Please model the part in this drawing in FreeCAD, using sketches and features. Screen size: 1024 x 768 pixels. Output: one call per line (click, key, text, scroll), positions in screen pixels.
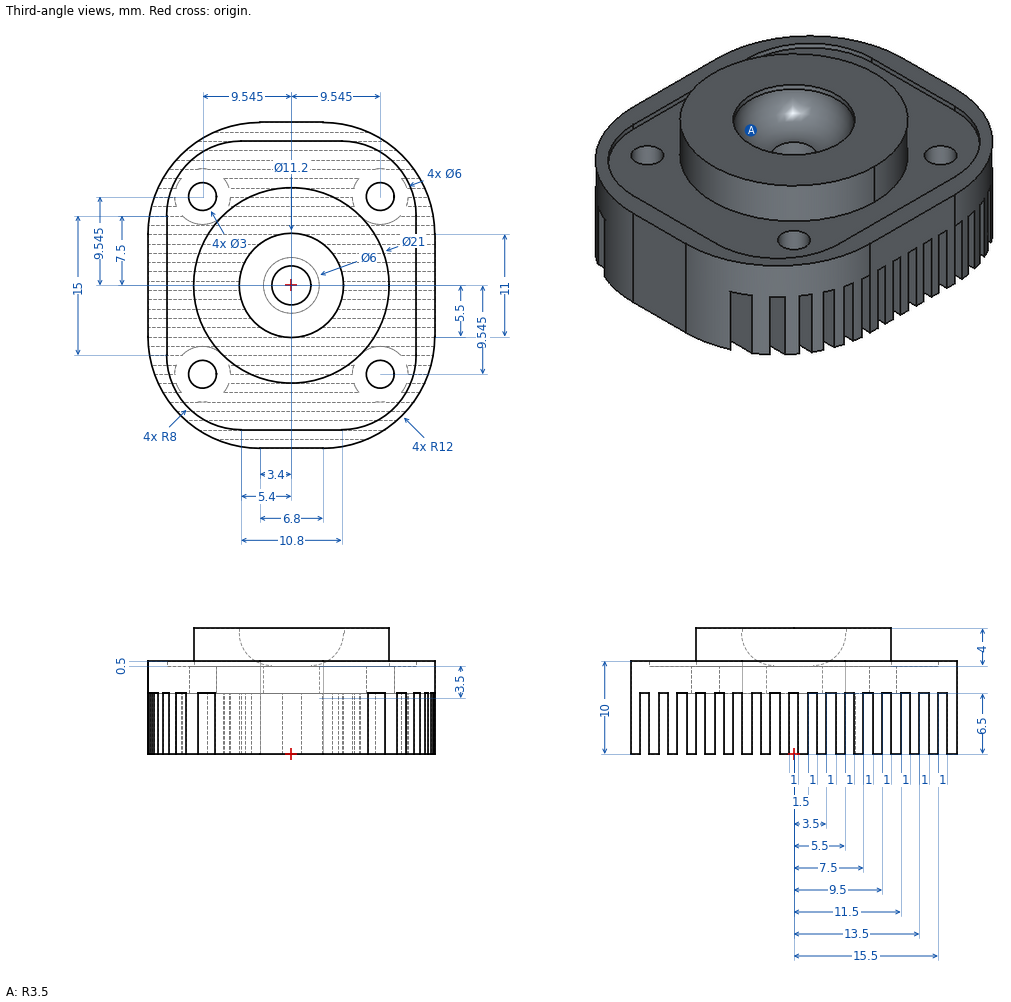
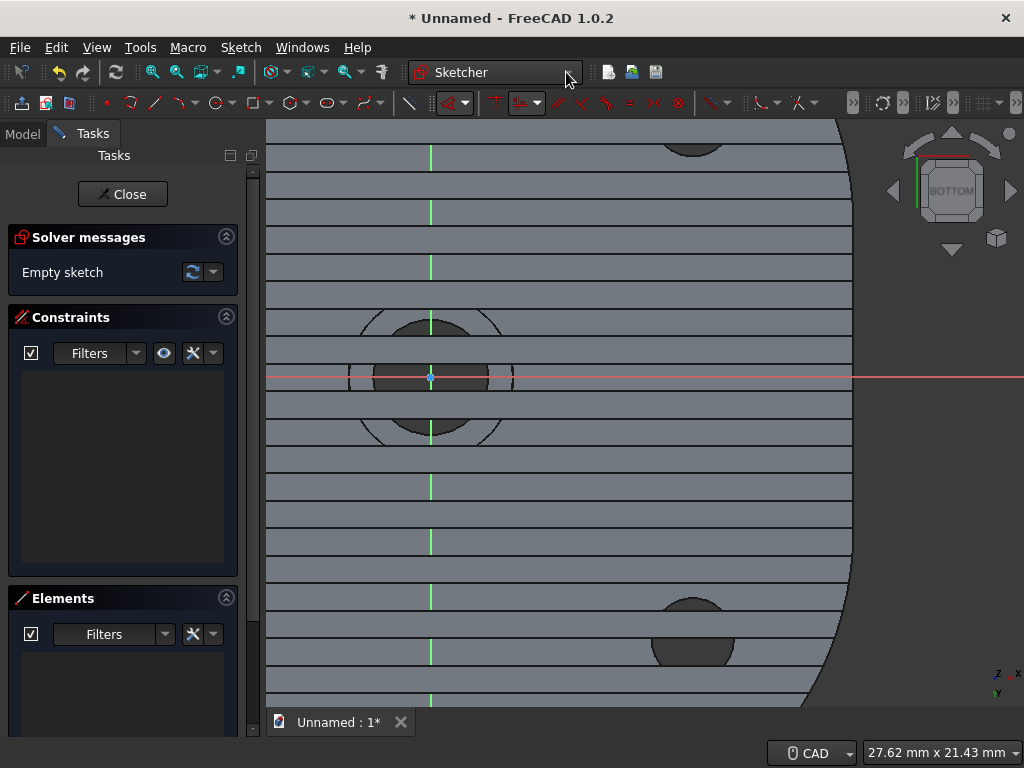
click(70, 104)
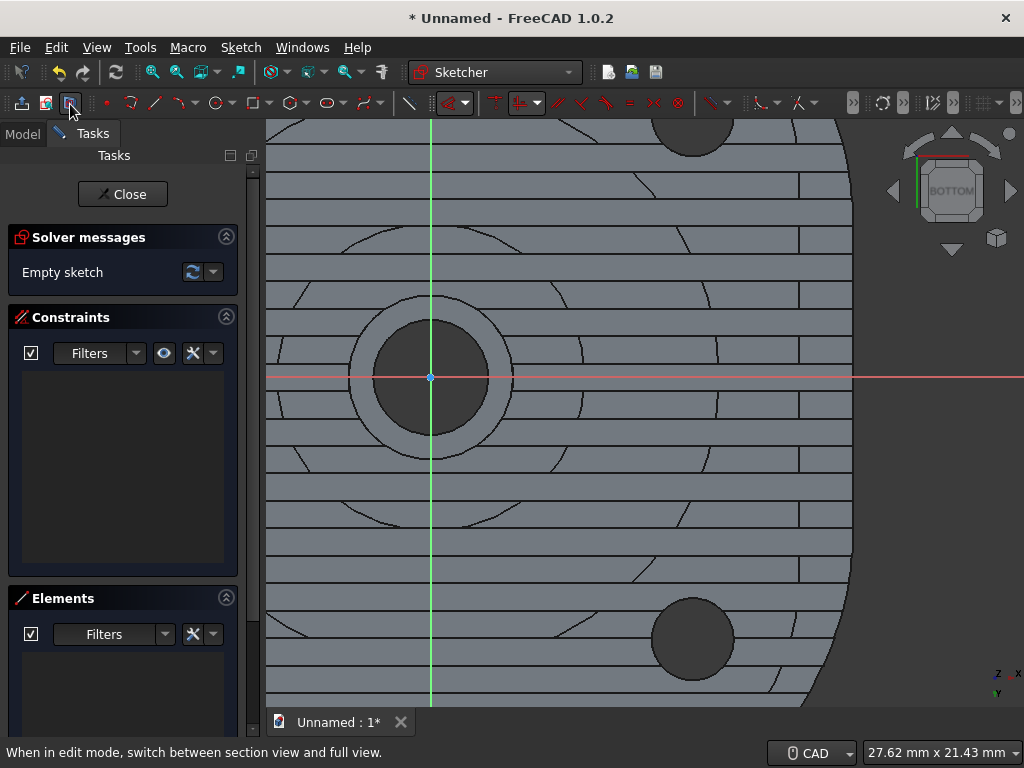
scroll(859, 574, down, 1)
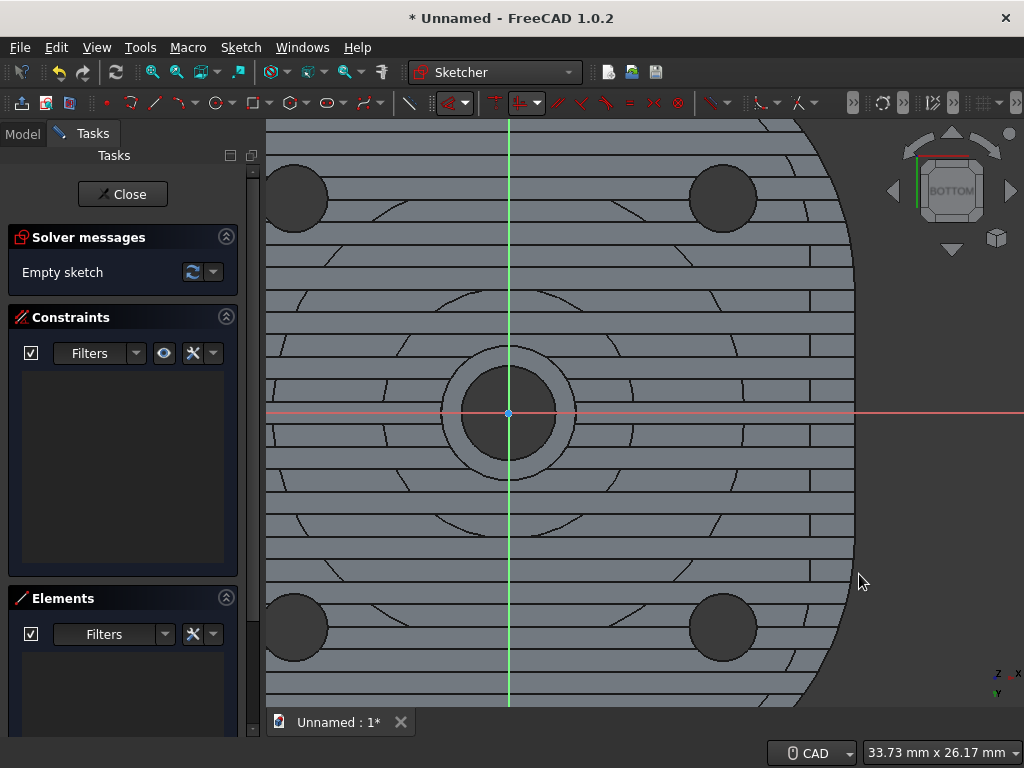
scroll(370, 413, up, 2)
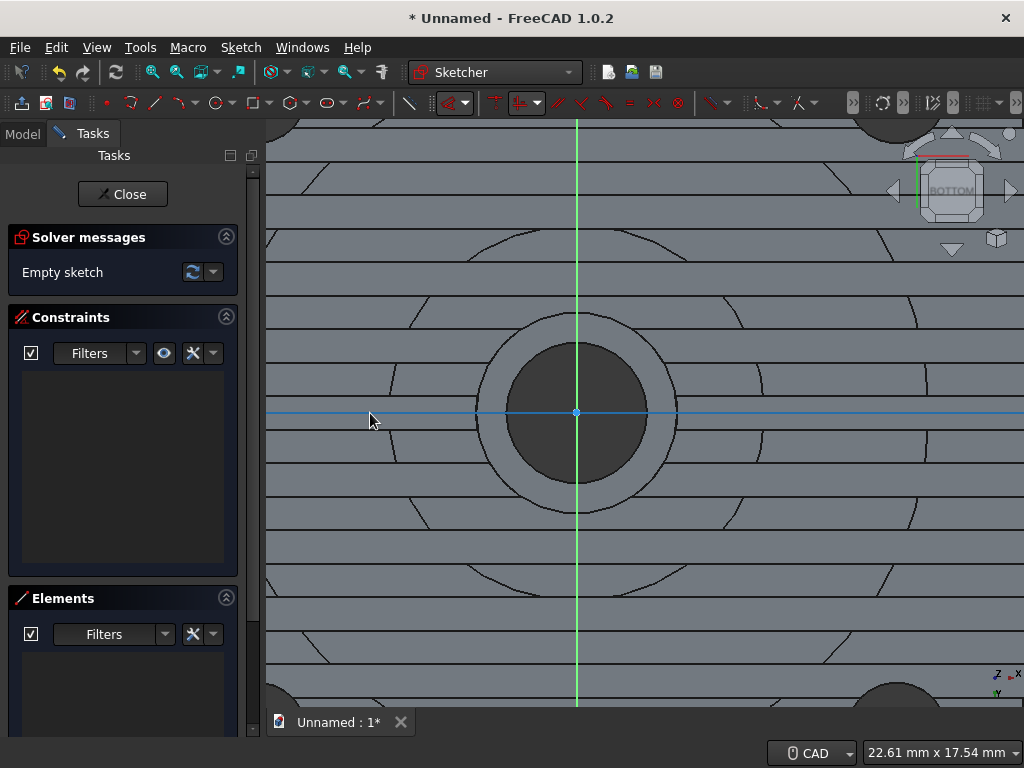
click(216, 104)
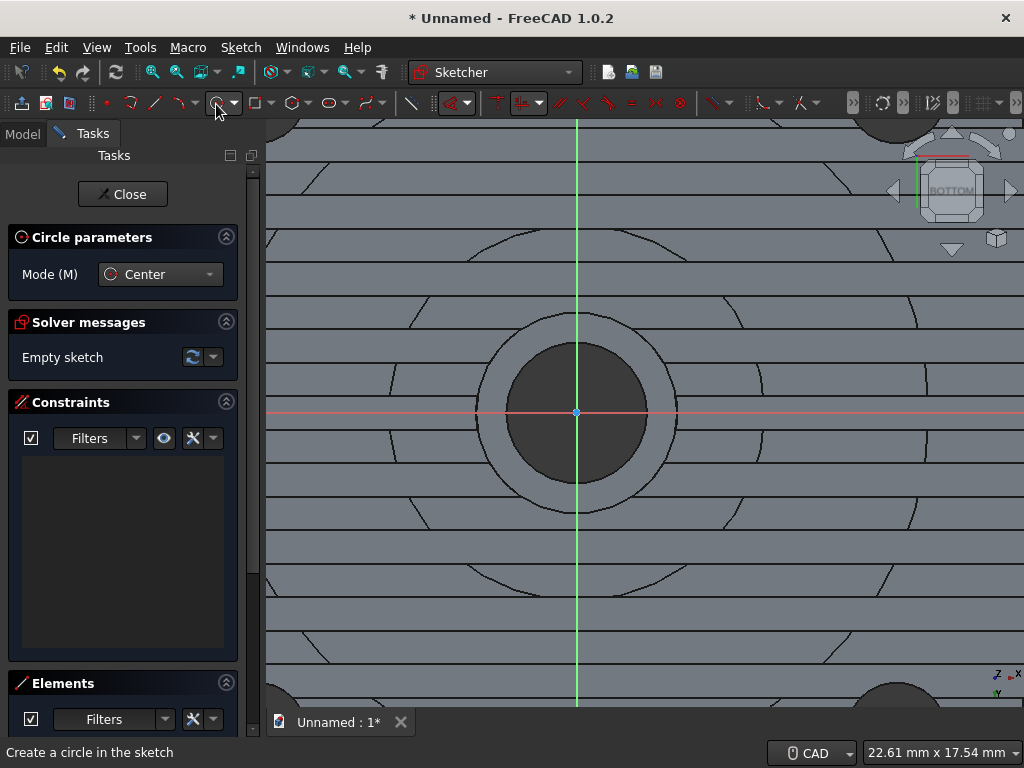
click(577, 413)
move(709, 280)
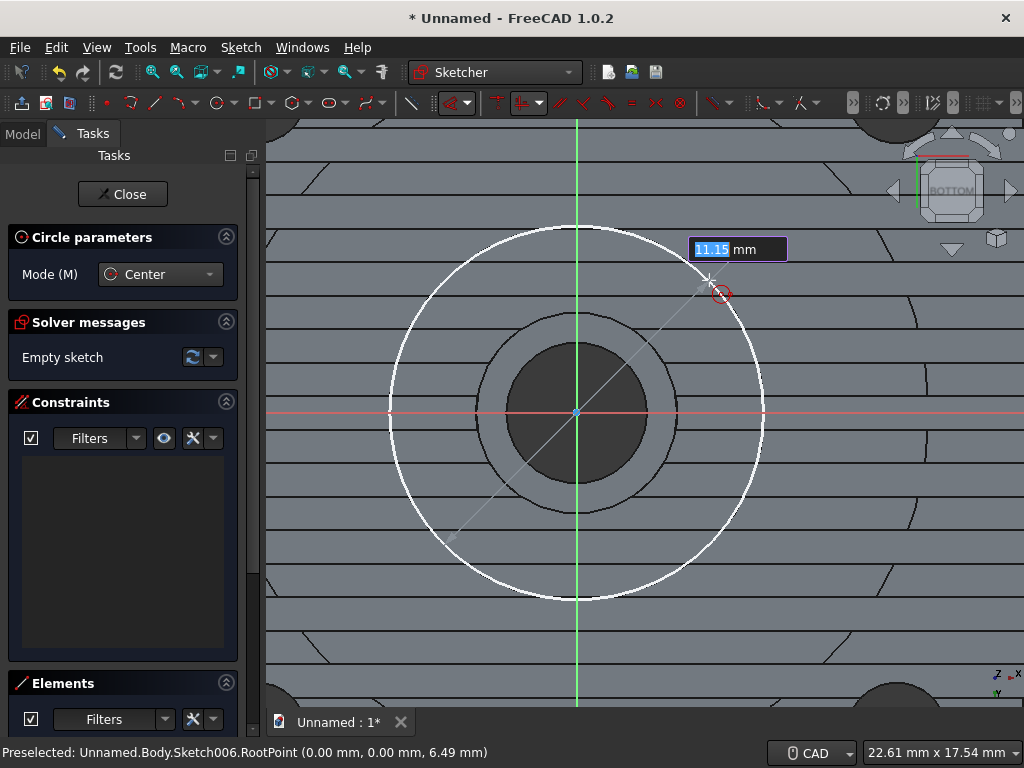
text(11.2)
key(Return)
key(Escape)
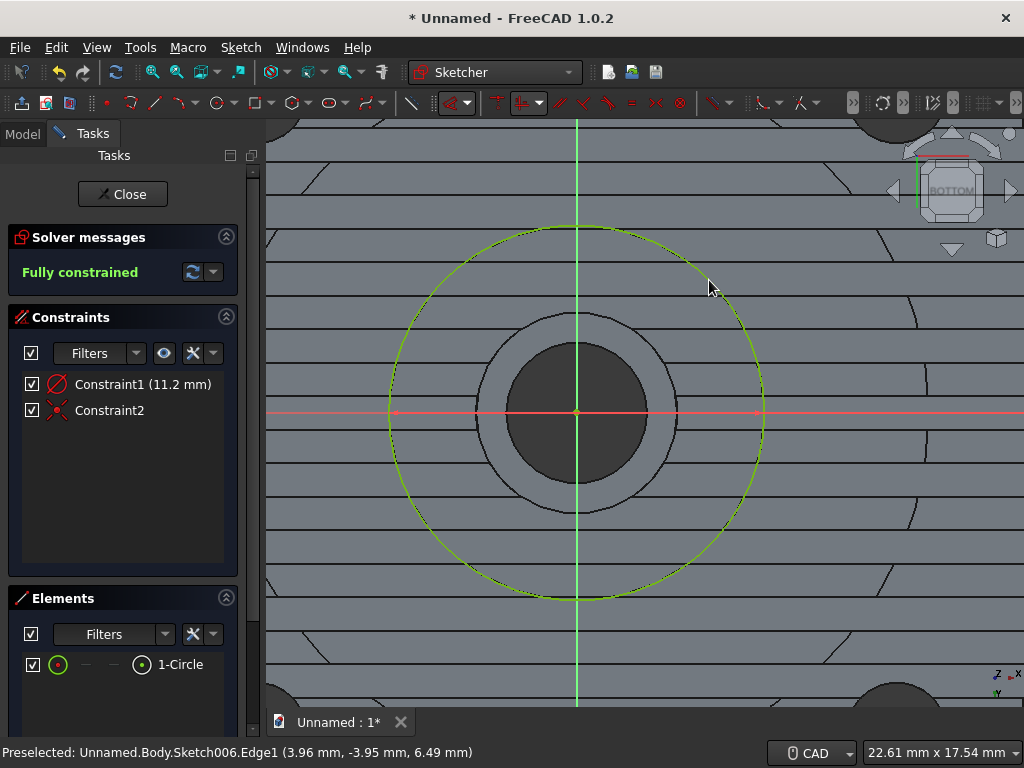
click(123, 194)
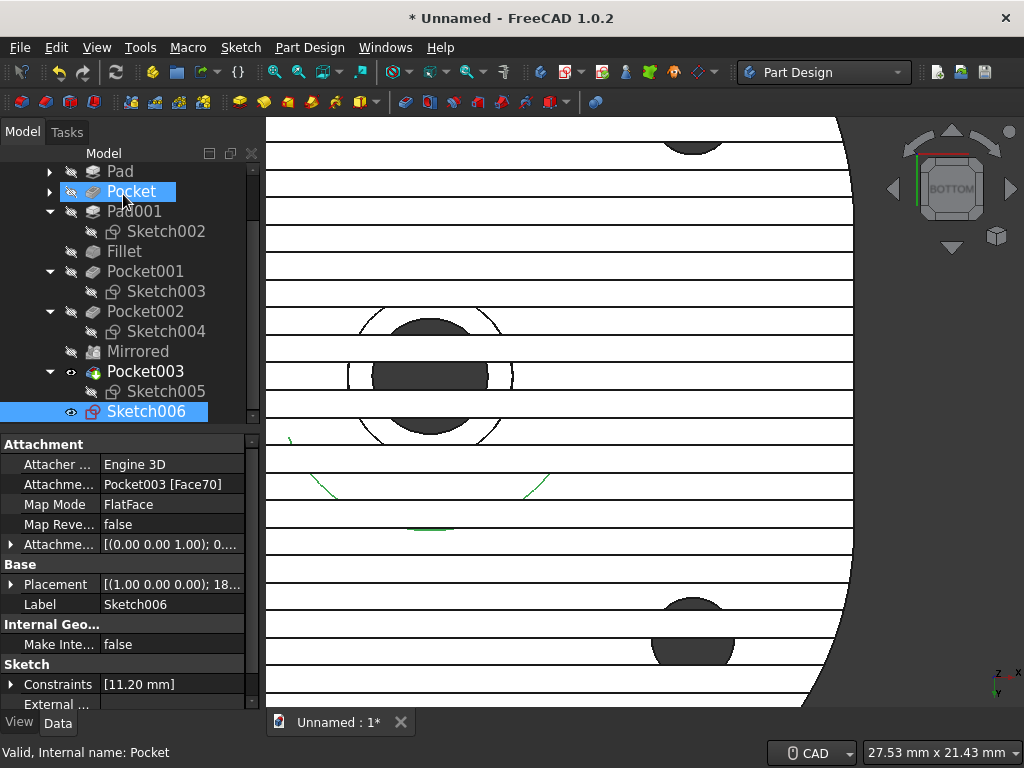
click(406, 102)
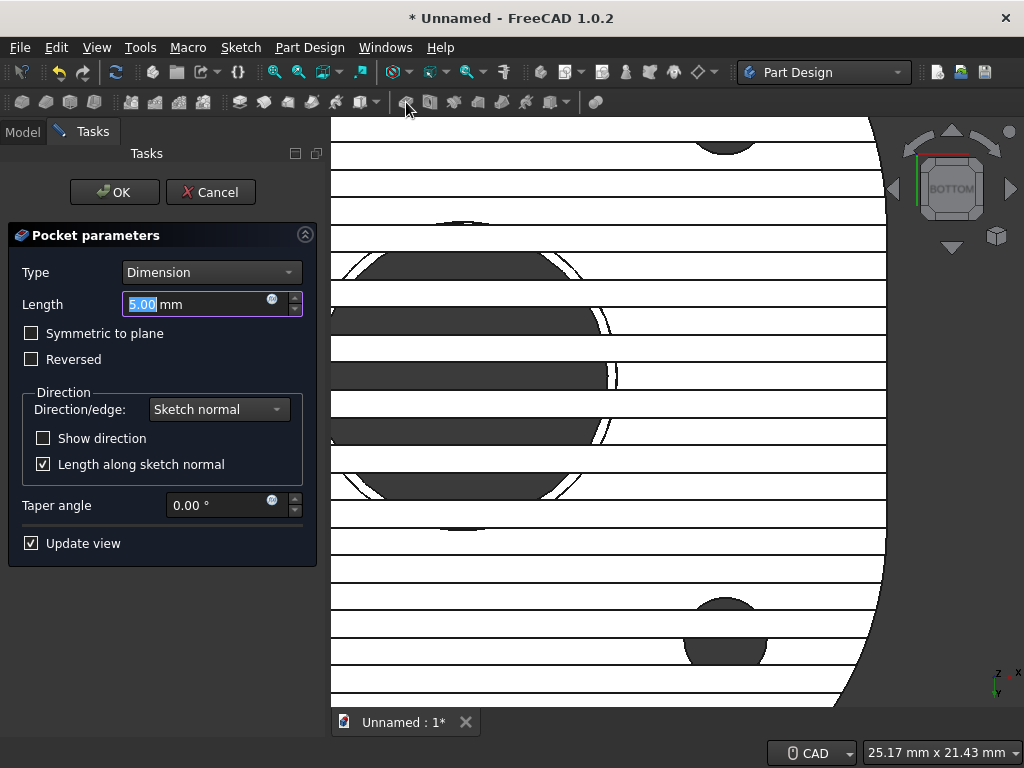
click(212, 272)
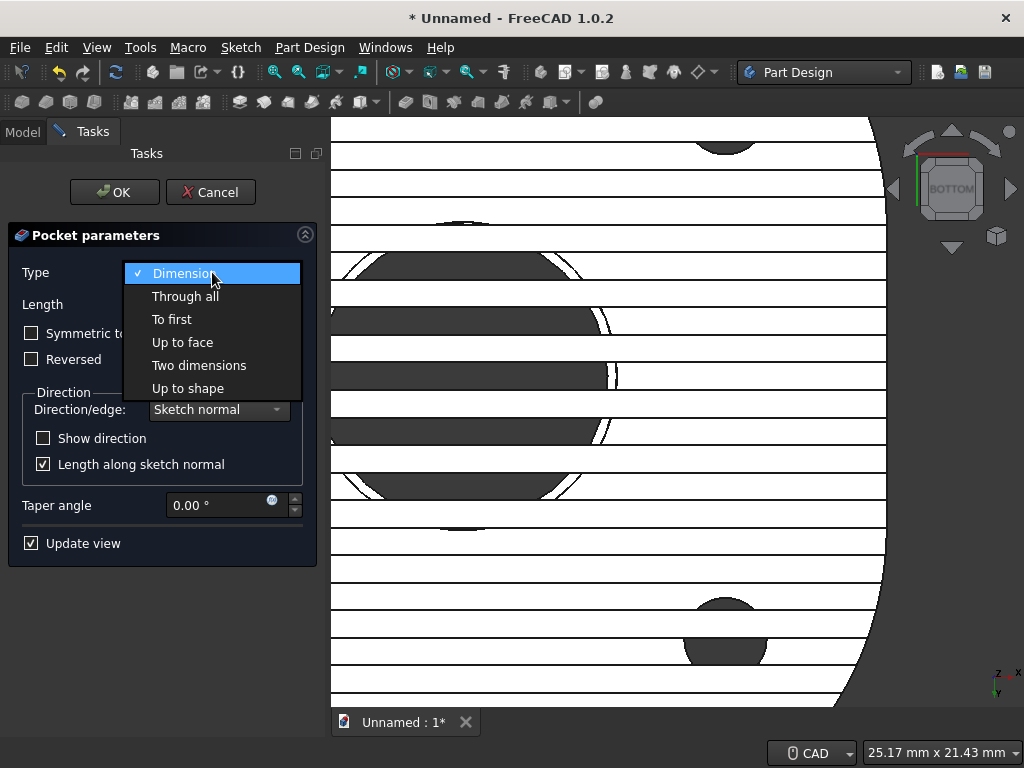
click(212, 296)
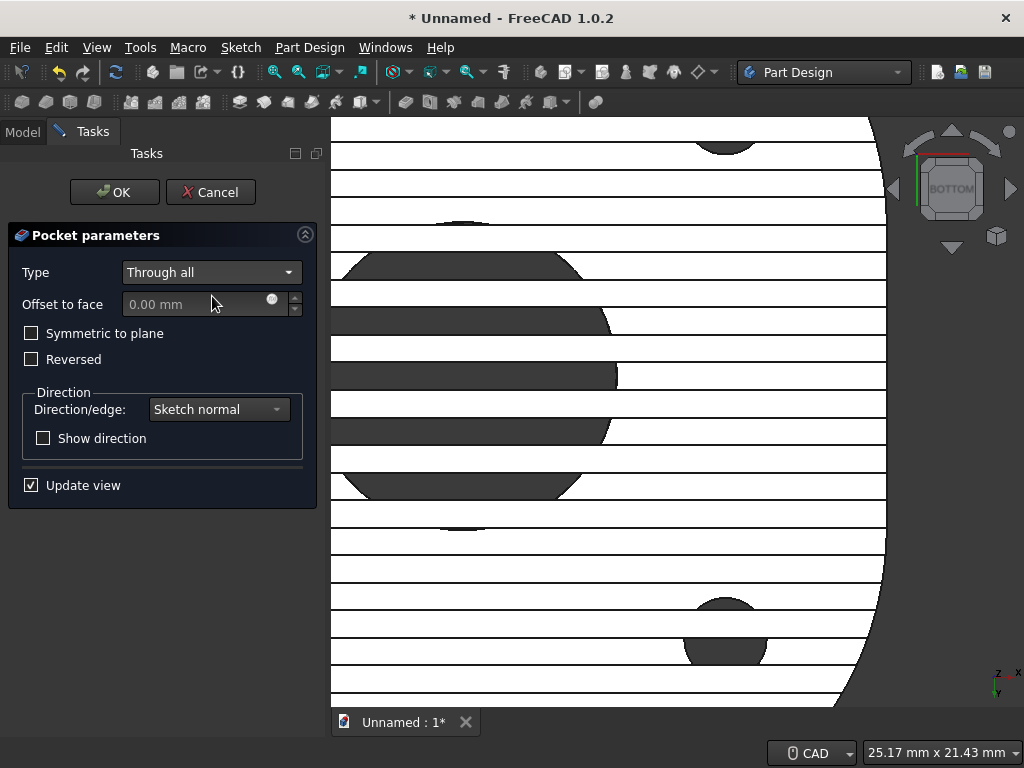
click(30, 359)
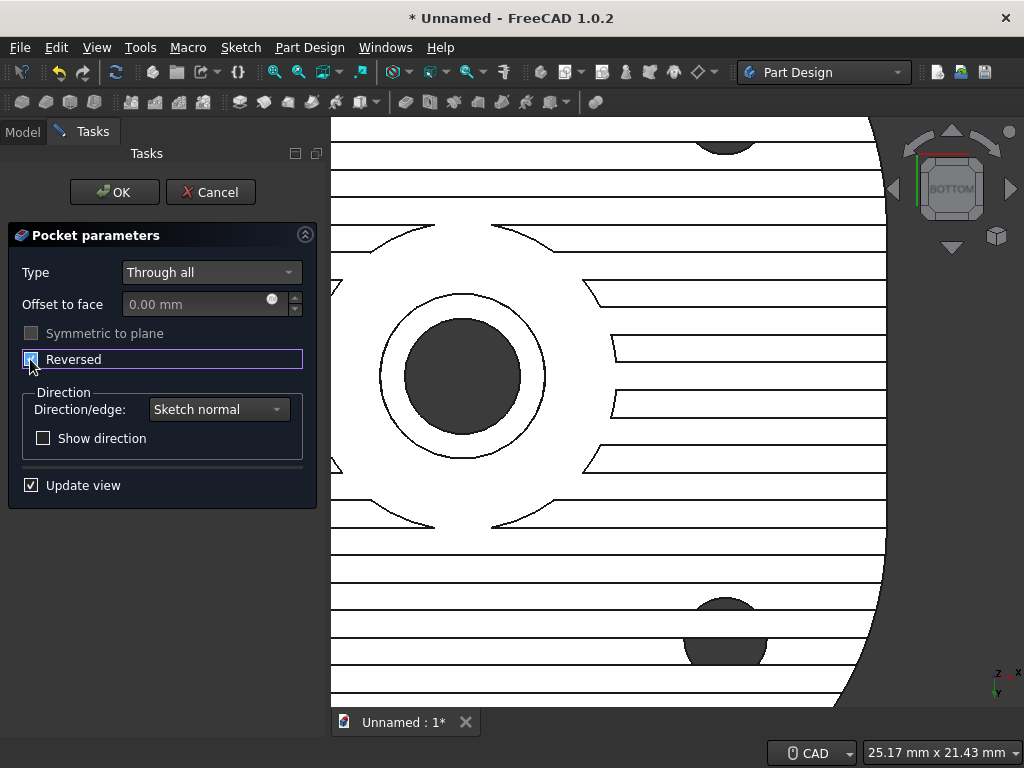
click(115, 192)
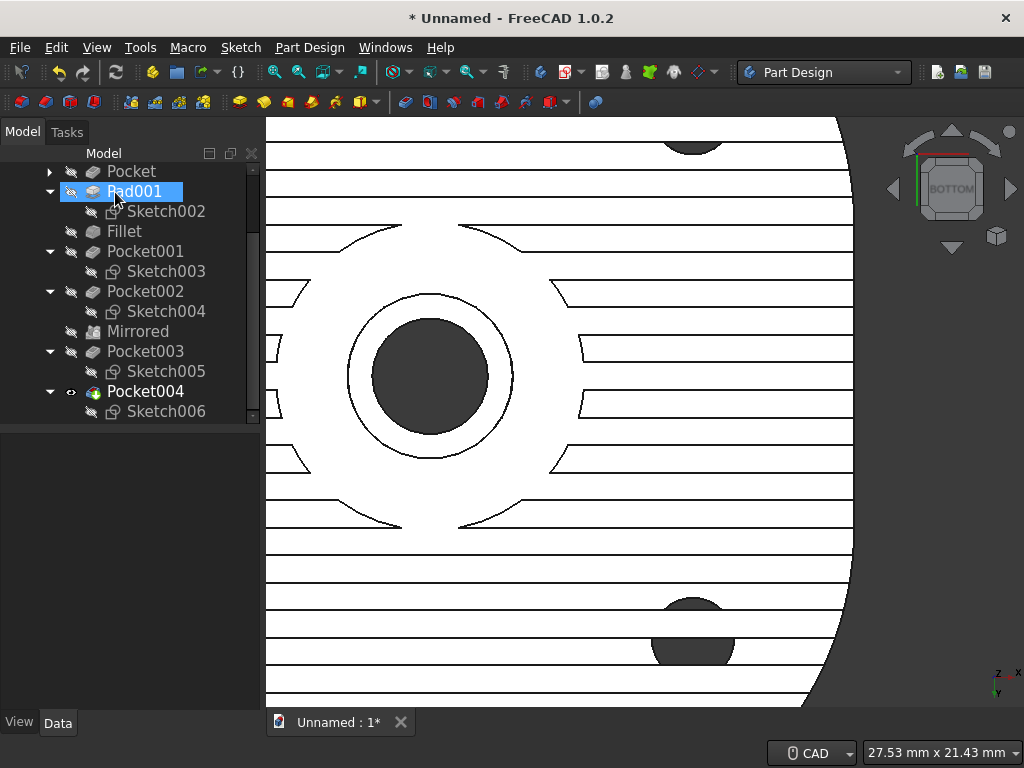
key(v)
key(f)